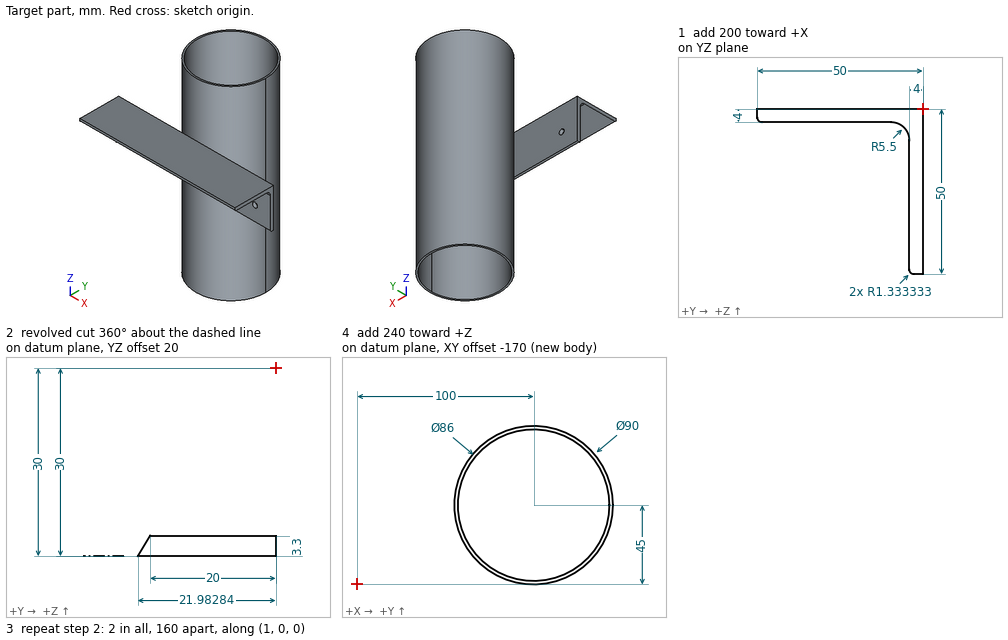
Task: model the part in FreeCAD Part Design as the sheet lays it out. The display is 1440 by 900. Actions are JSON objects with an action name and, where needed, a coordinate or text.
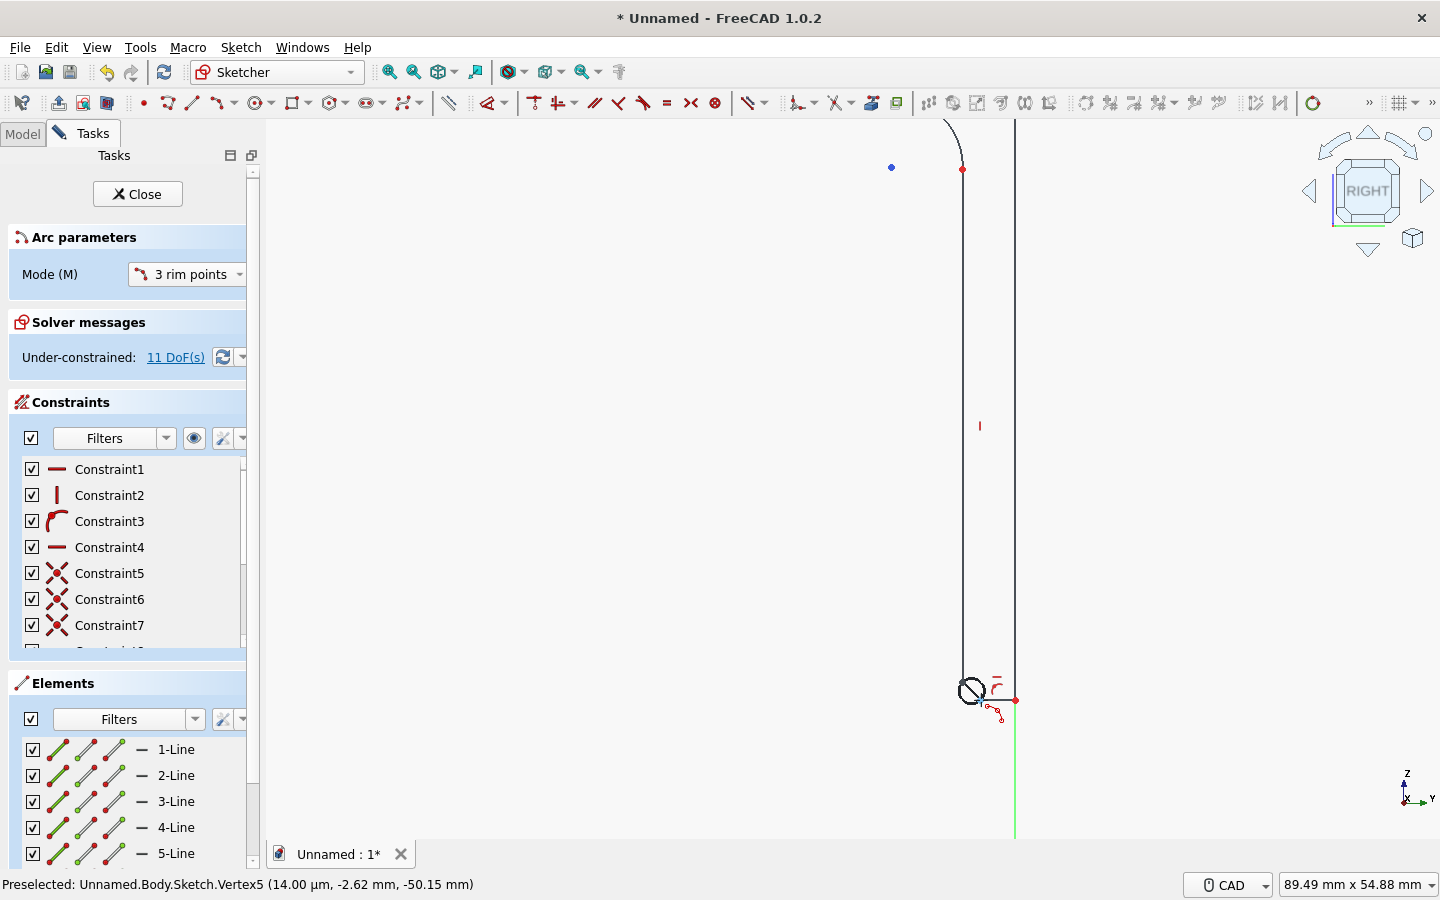
{"action": "scroll", "coordinate": [968, 693], "scroll_direction": "up", "scroll_amount": 6}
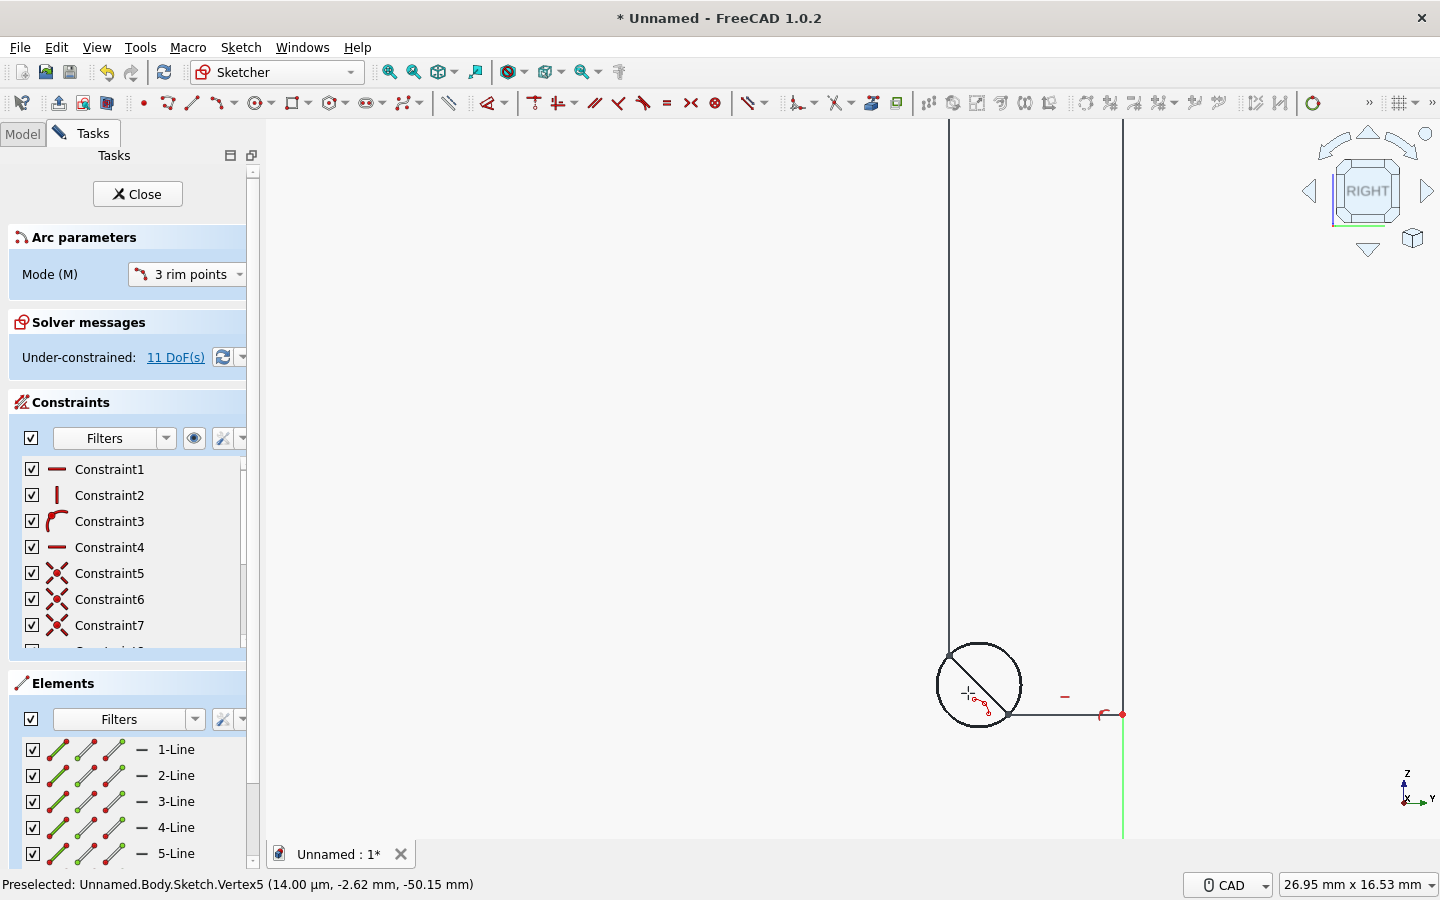
{"action": "left_click", "coordinate": [966, 691]}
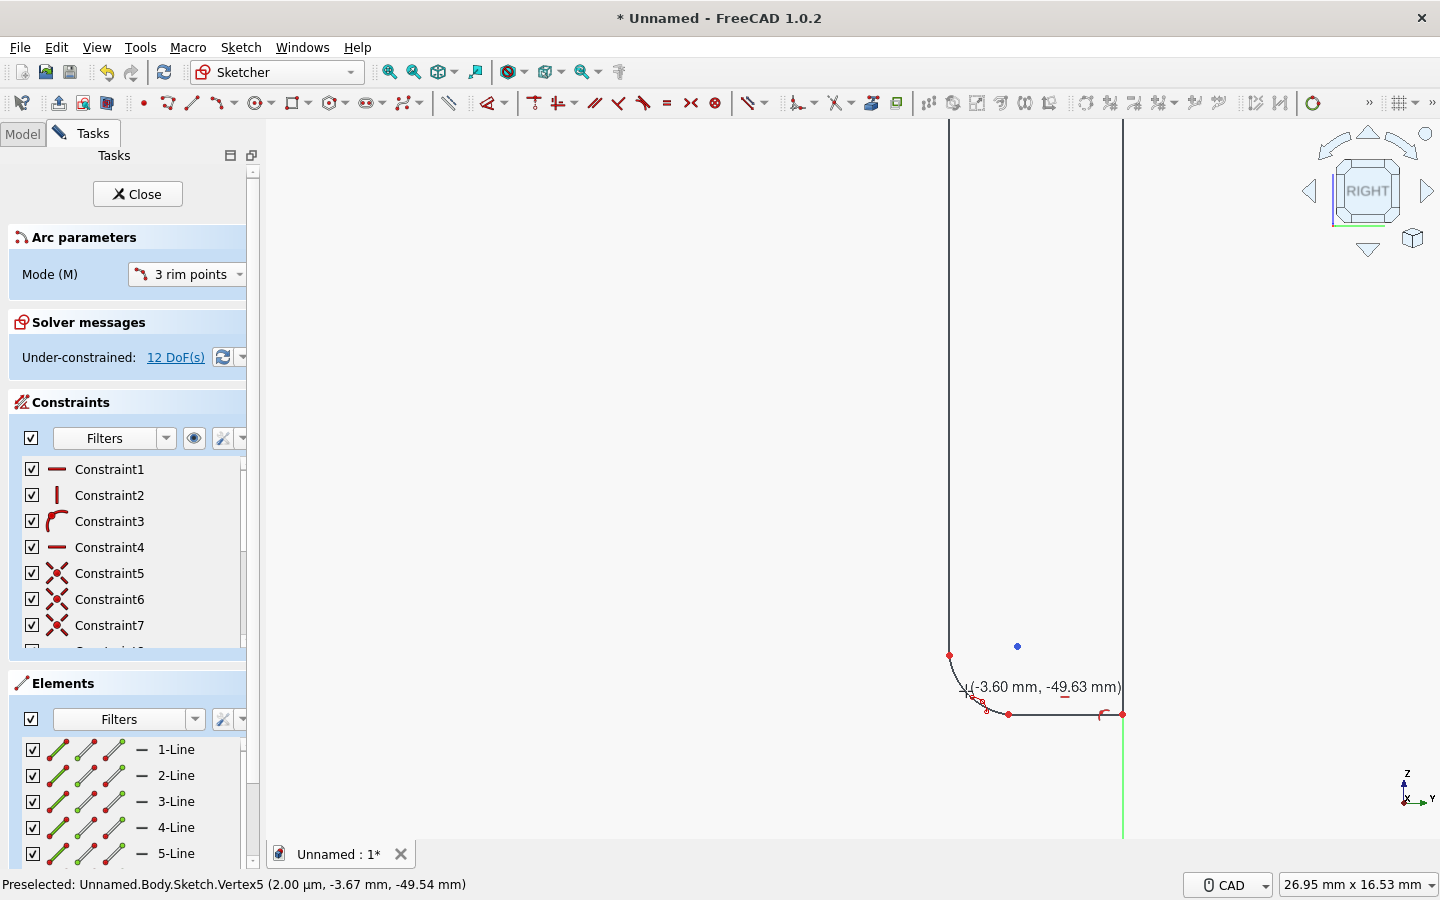
{"action": "scroll", "coordinate": [974, 697], "scroll_direction": "down", "scroll_amount": 8}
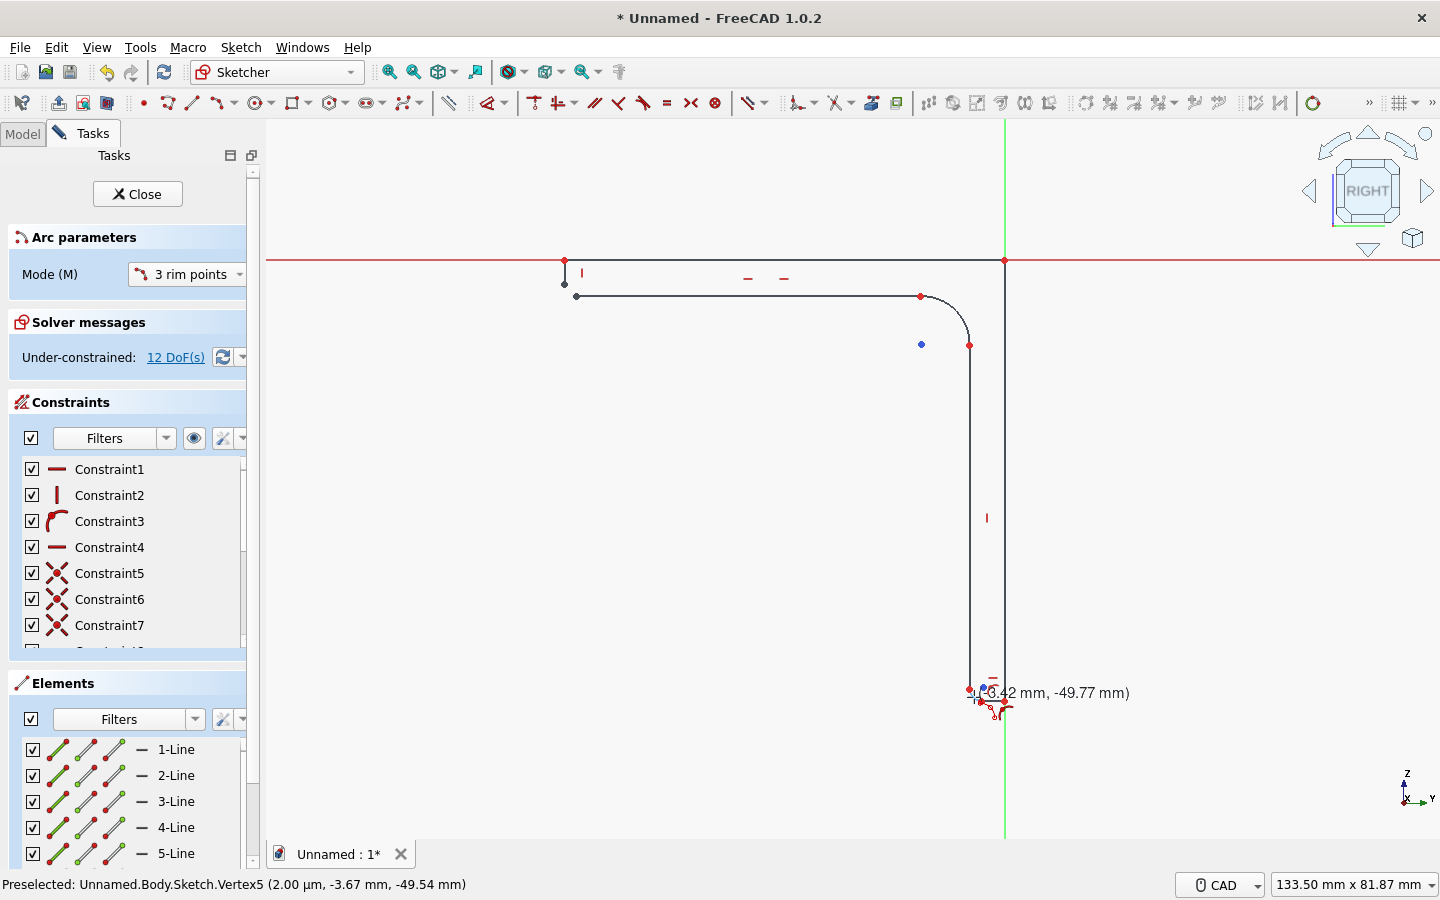
{"action": "scroll", "coordinate": [565, 284], "scroll_direction": "up", "scroll_amount": 2}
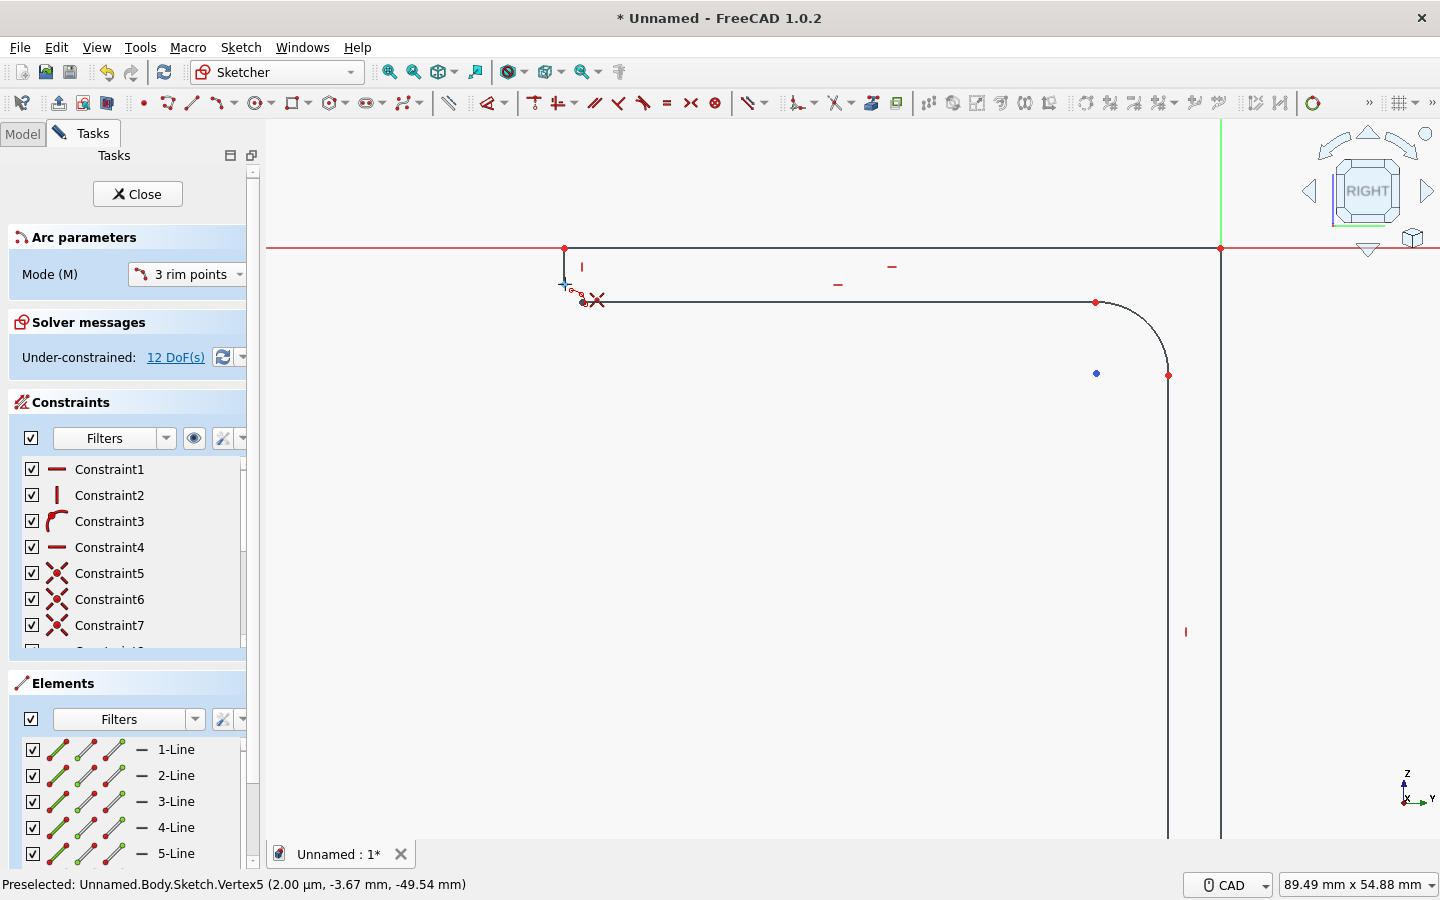
{"action": "left_click", "coordinate": [564, 284]}
{"action": "left_click", "coordinate": [582, 302]}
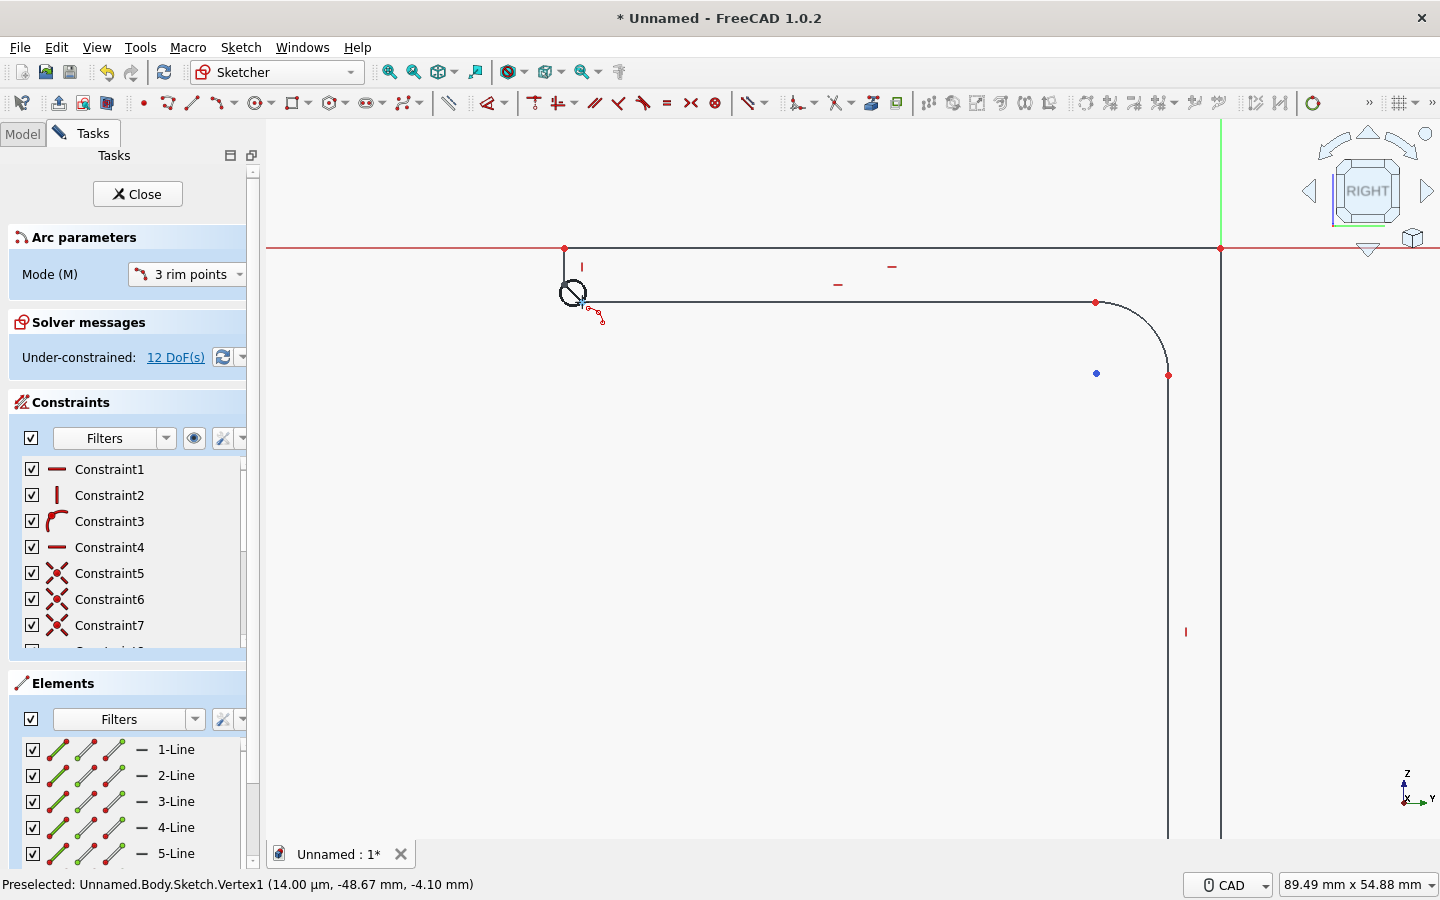
{"action": "scroll", "coordinate": [570, 296], "scroll_direction": "up", "scroll_amount": 6}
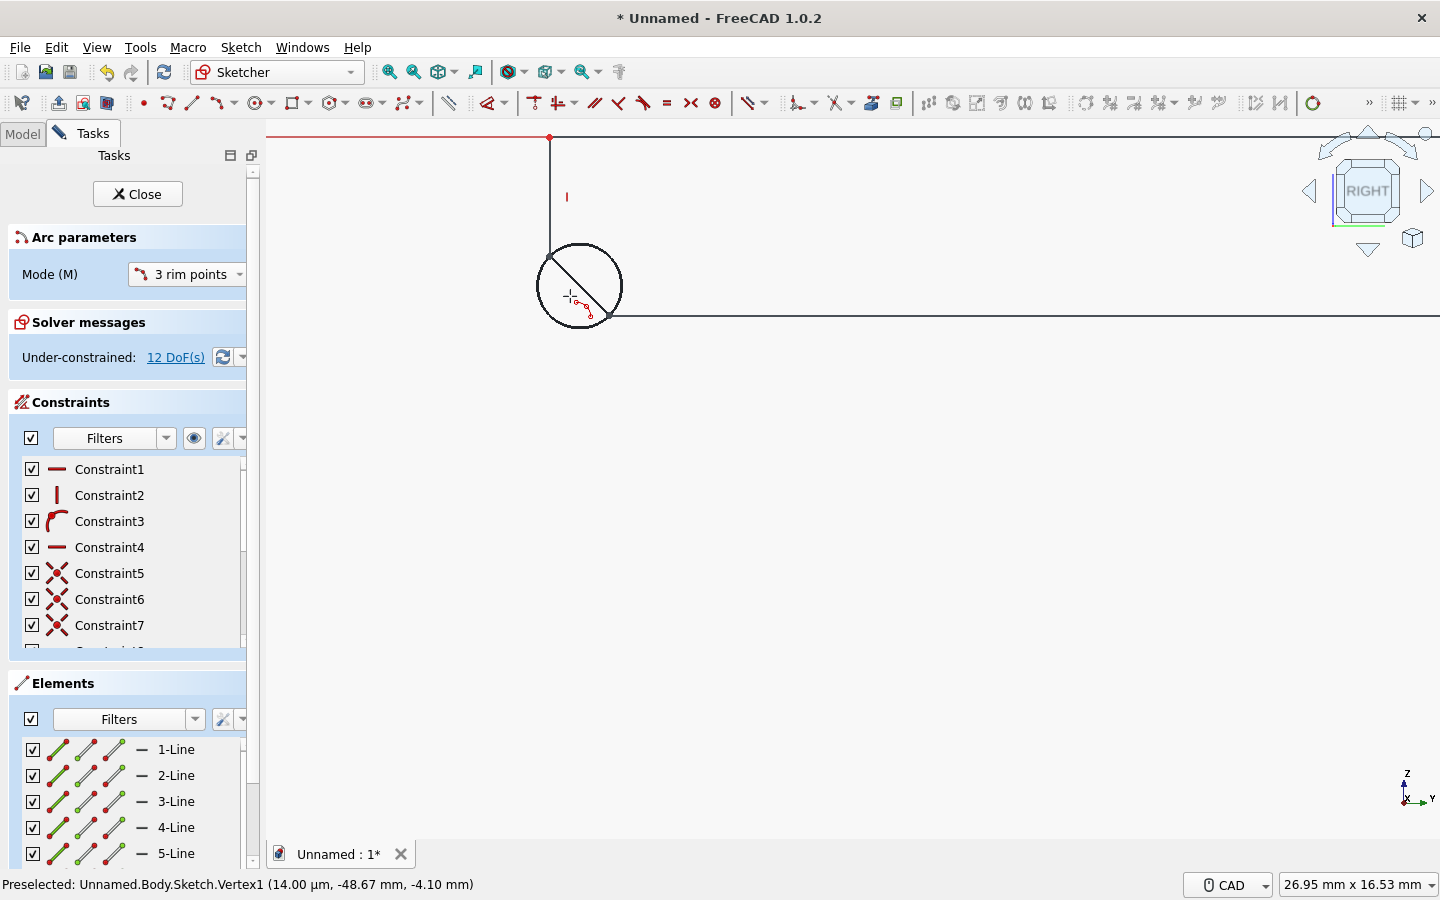
{"action": "left_click", "coordinate": [569, 294]}
{"action": "key", "text": "Escape"}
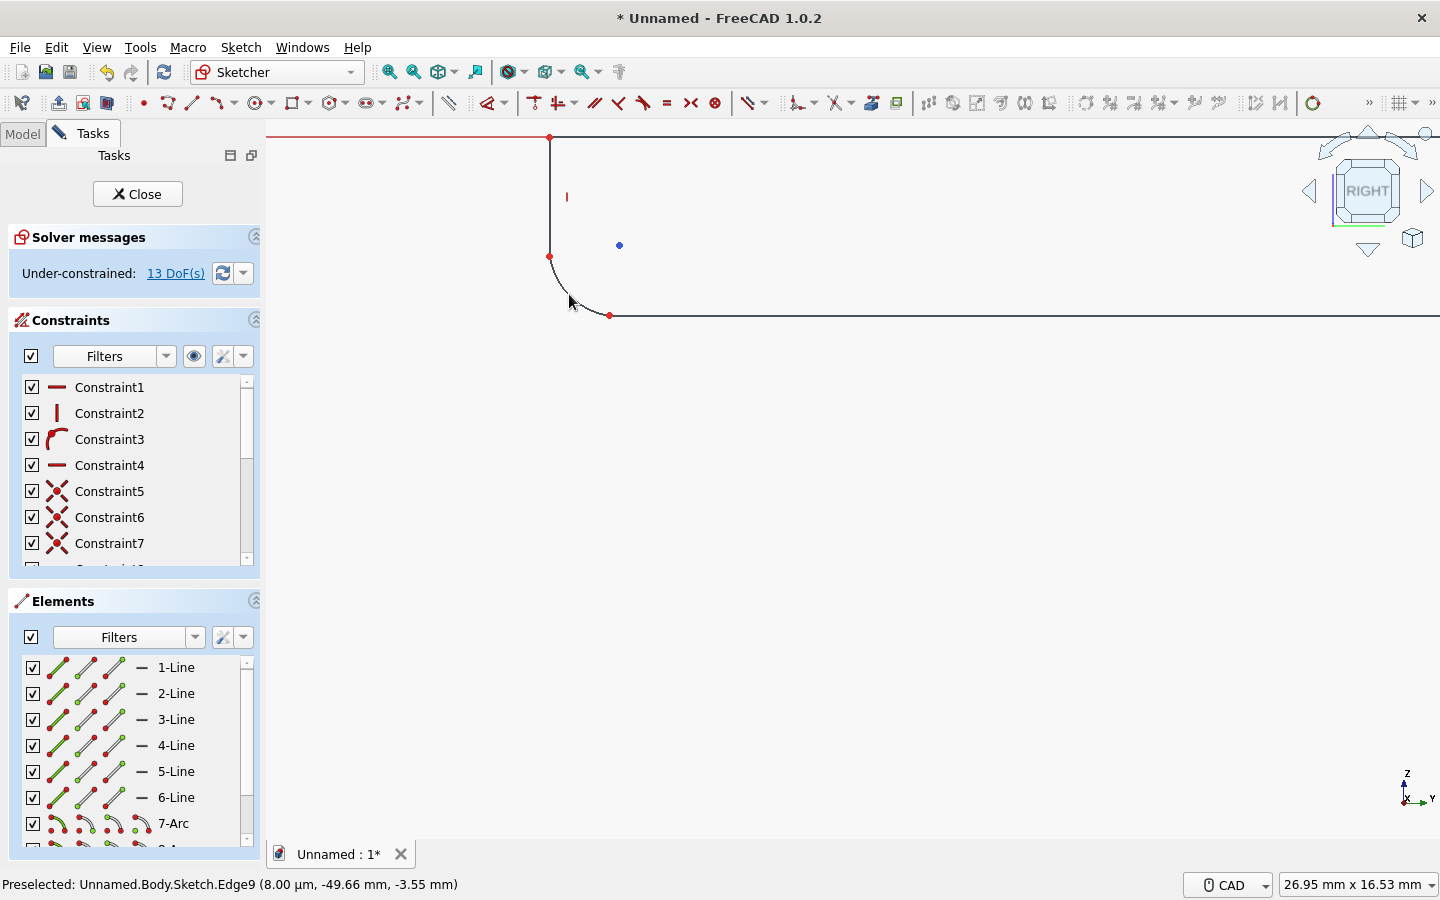
{"action": "scroll", "coordinate": [568, 290], "scroll_direction": "down", "scroll_amount": 8}